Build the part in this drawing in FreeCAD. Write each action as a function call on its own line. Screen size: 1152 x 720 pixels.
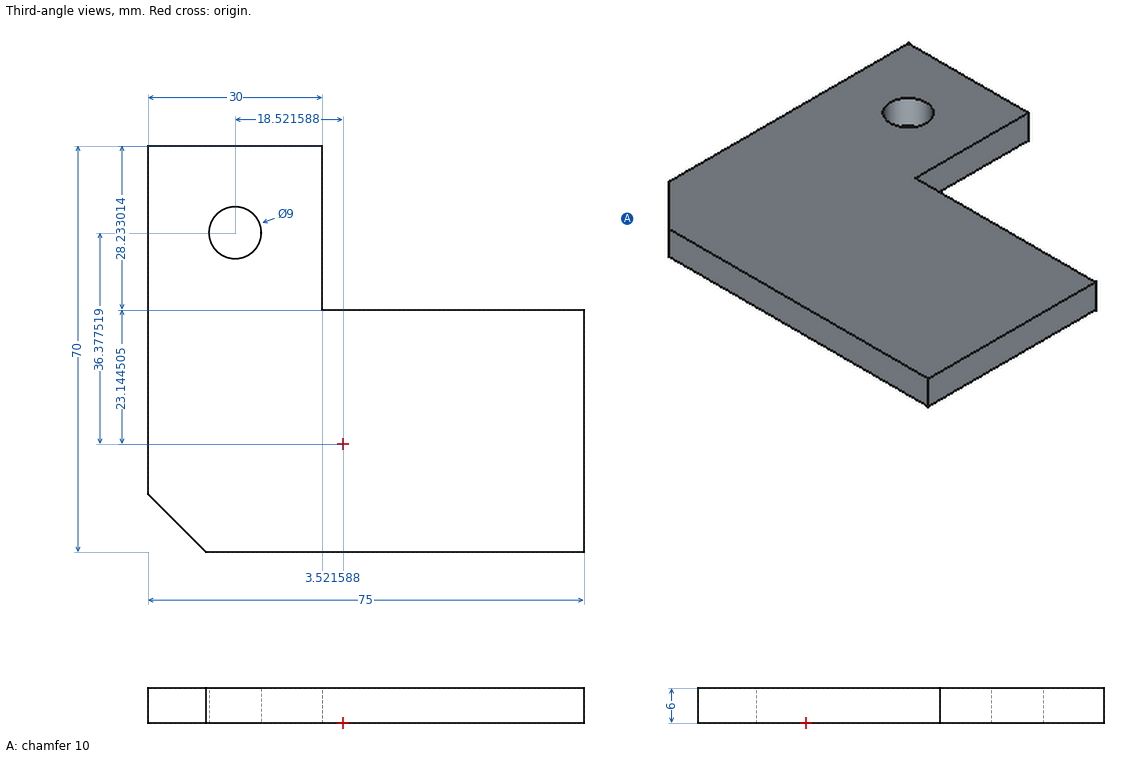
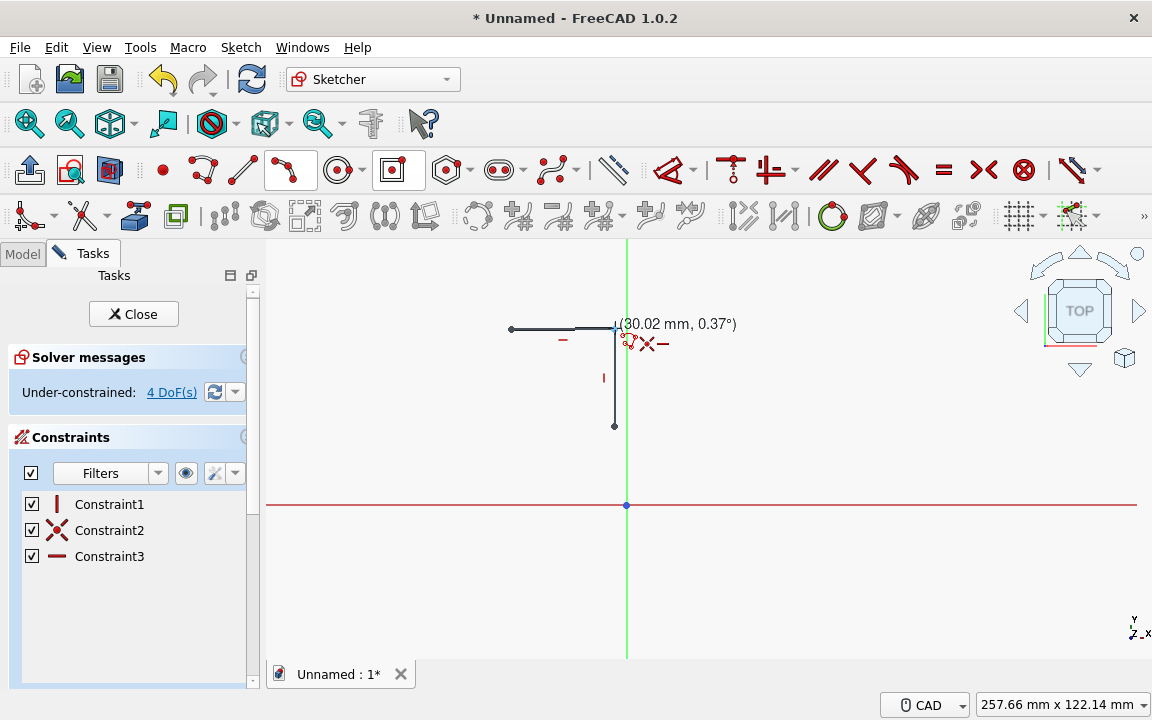
click(512, 569)
click(769, 569)
click(769, 426)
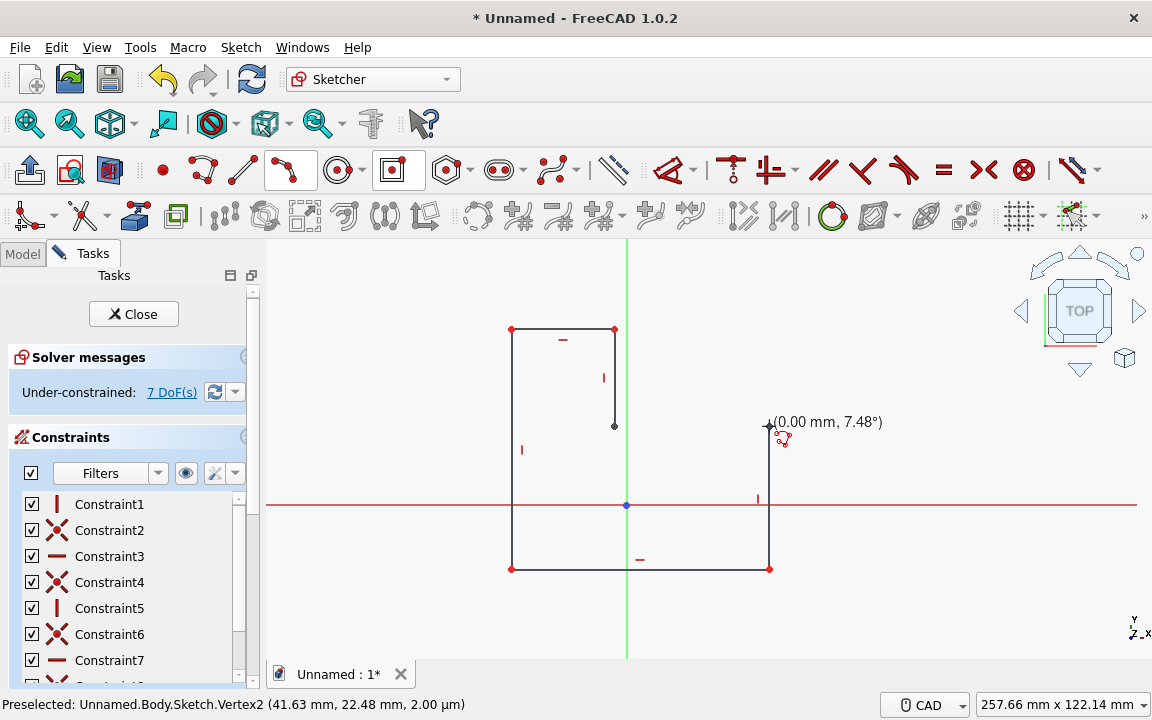
scroll(615, 426, up, 2)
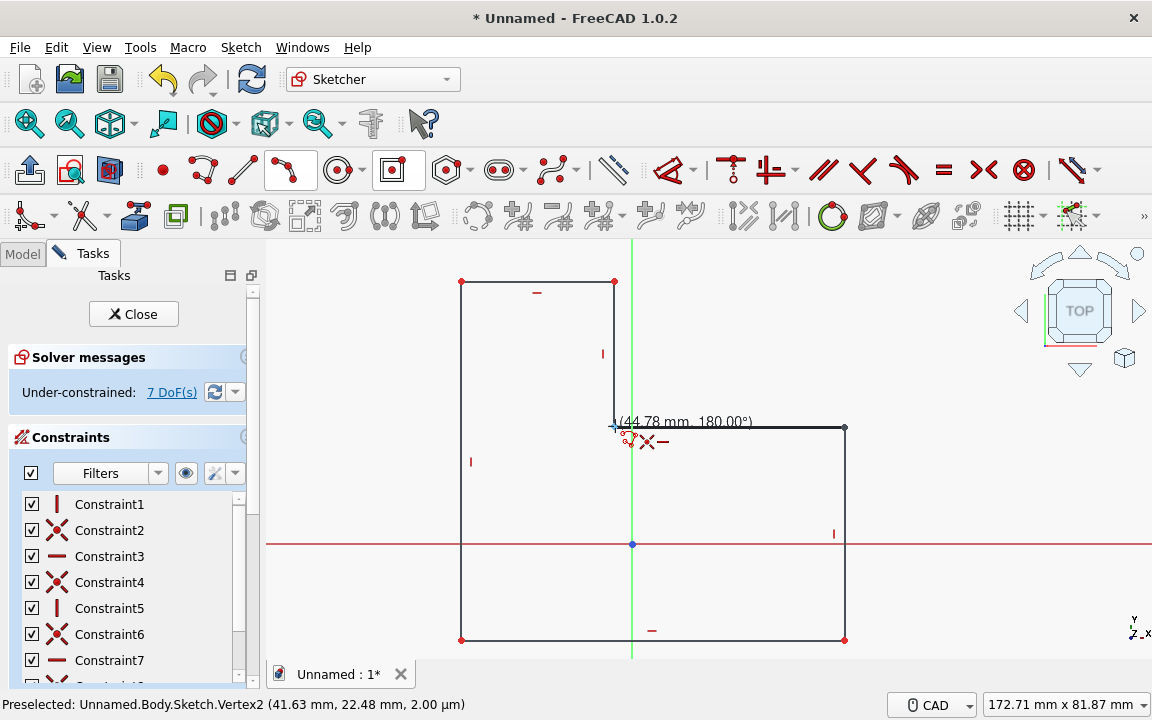
click(614, 426)
key(Escape)
key(Escape)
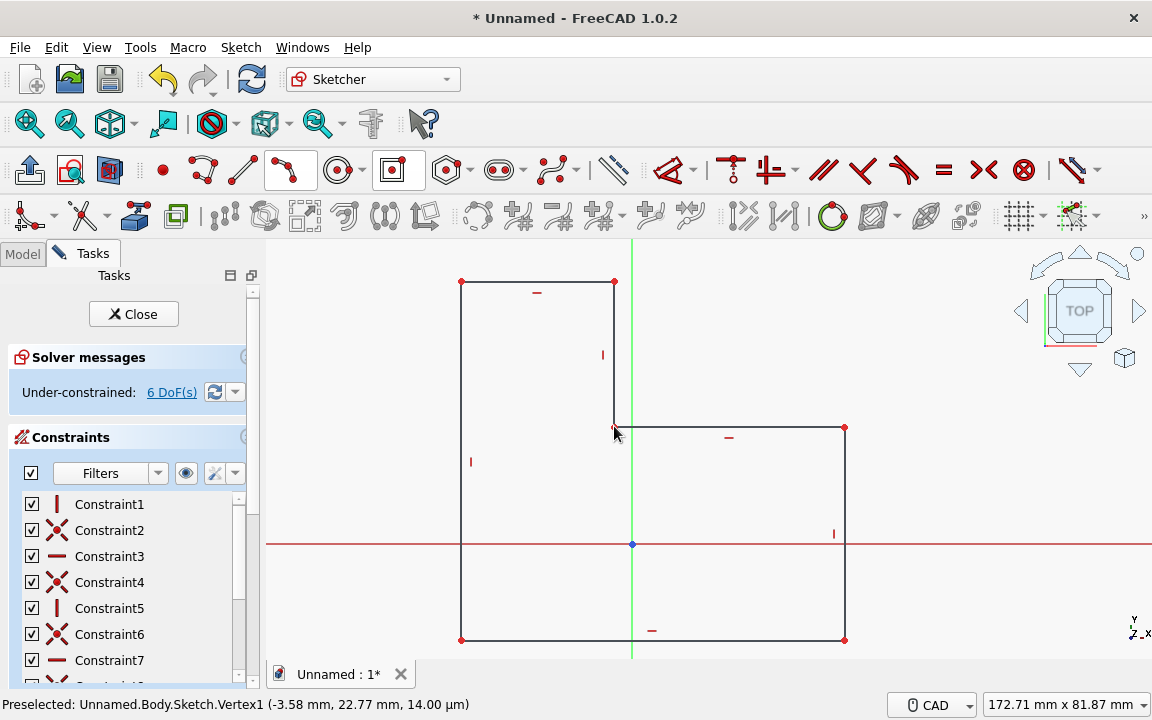
click(568, 282)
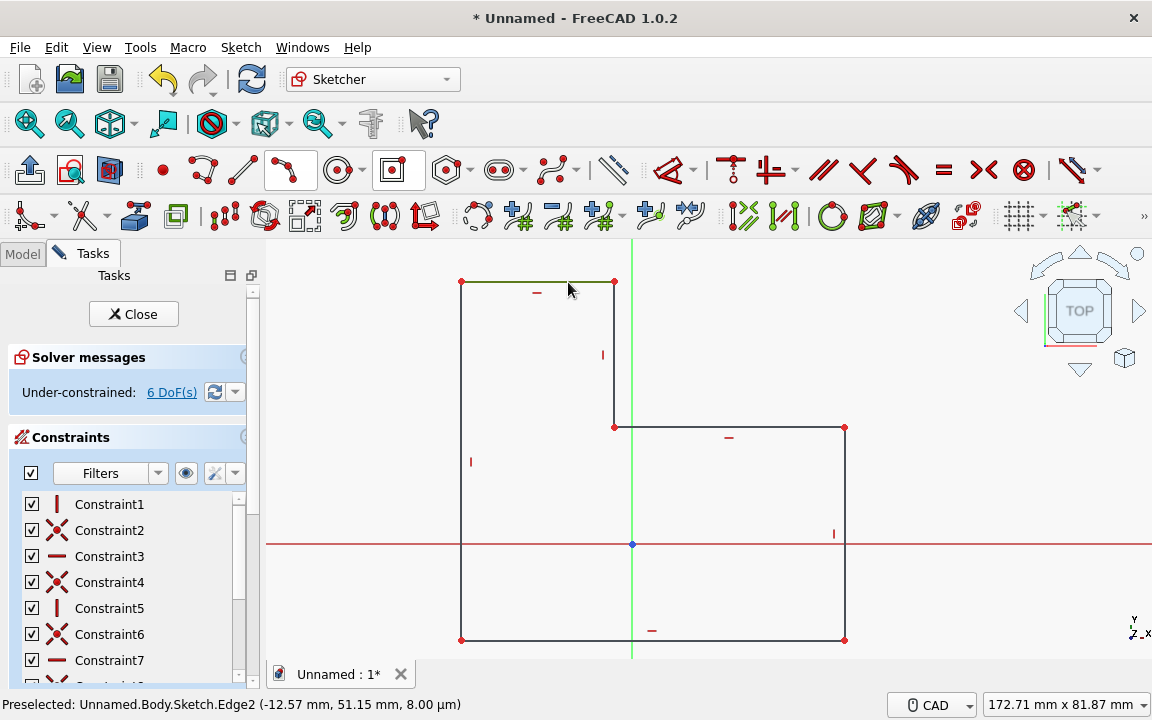
click(696, 170)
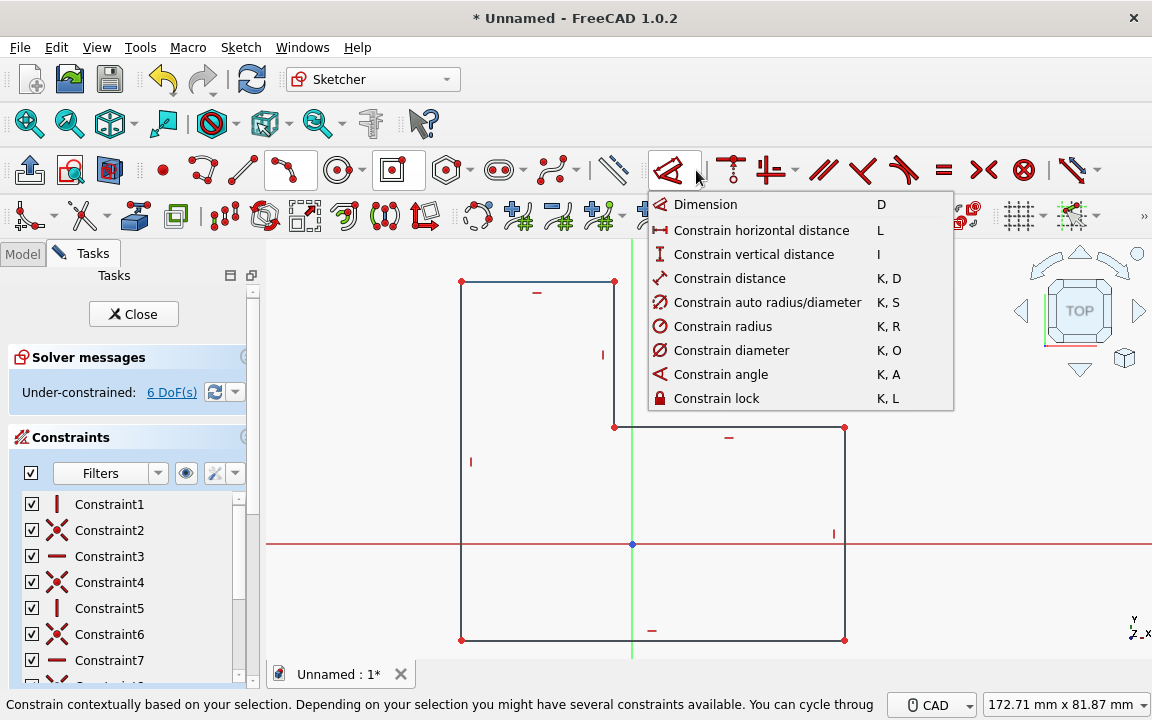
click(801, 230)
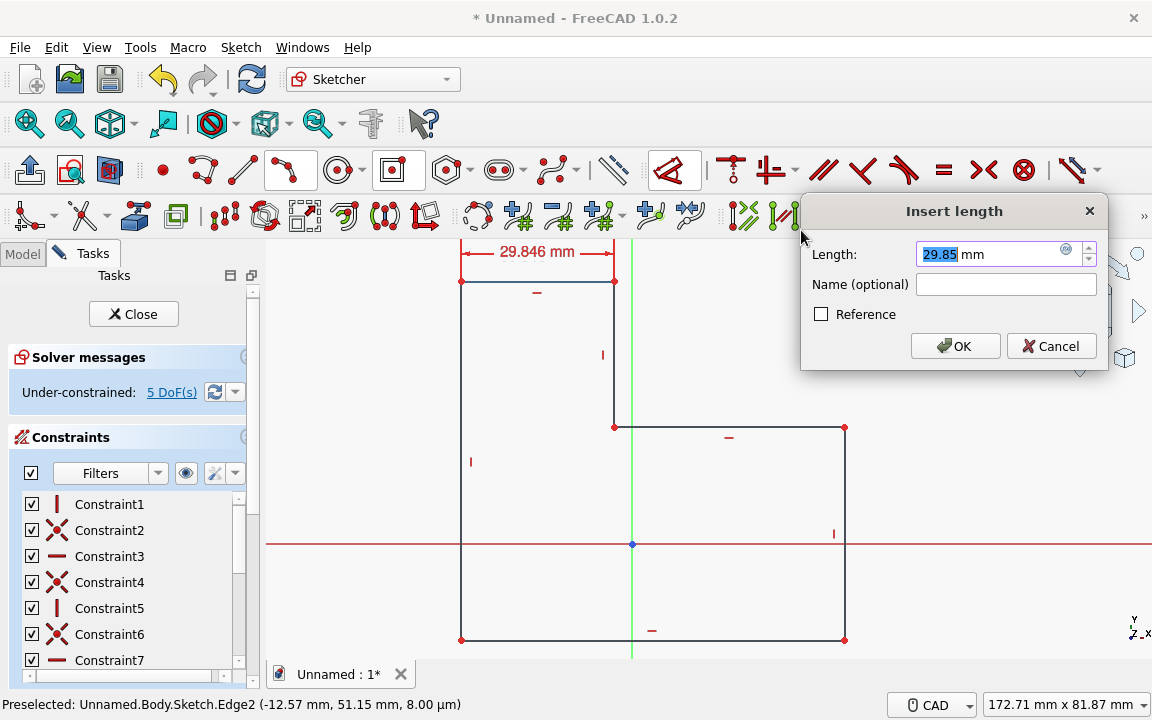
text(30)
key(Return)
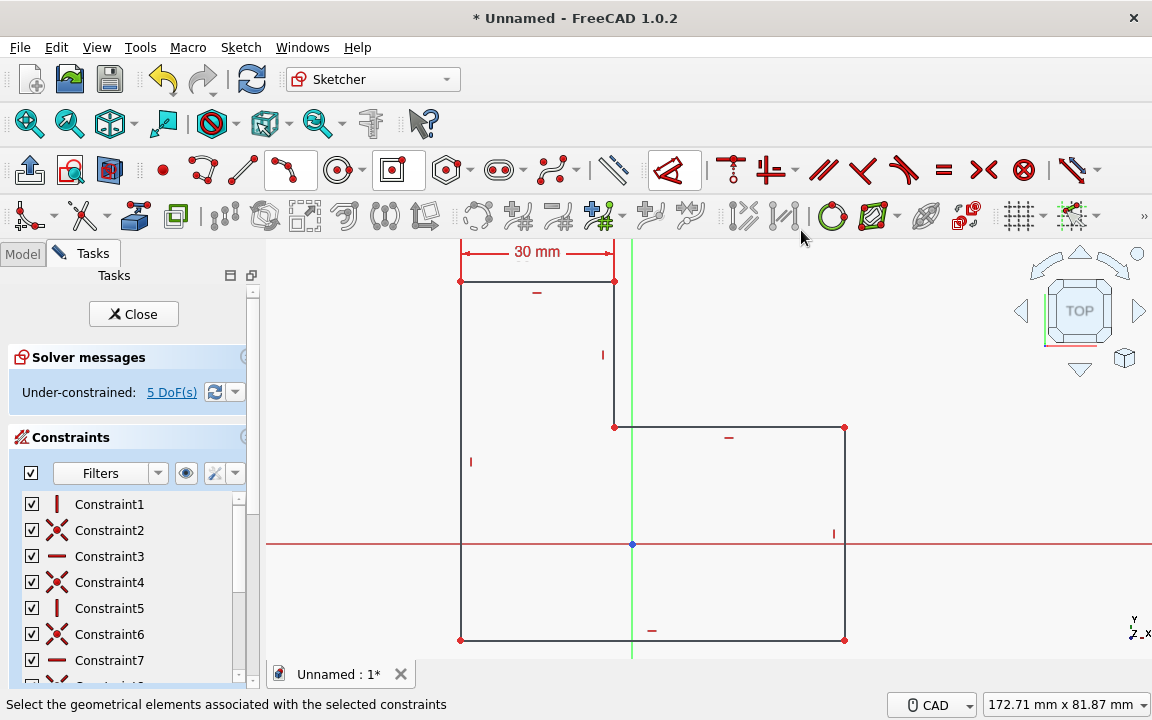
click(461, 389)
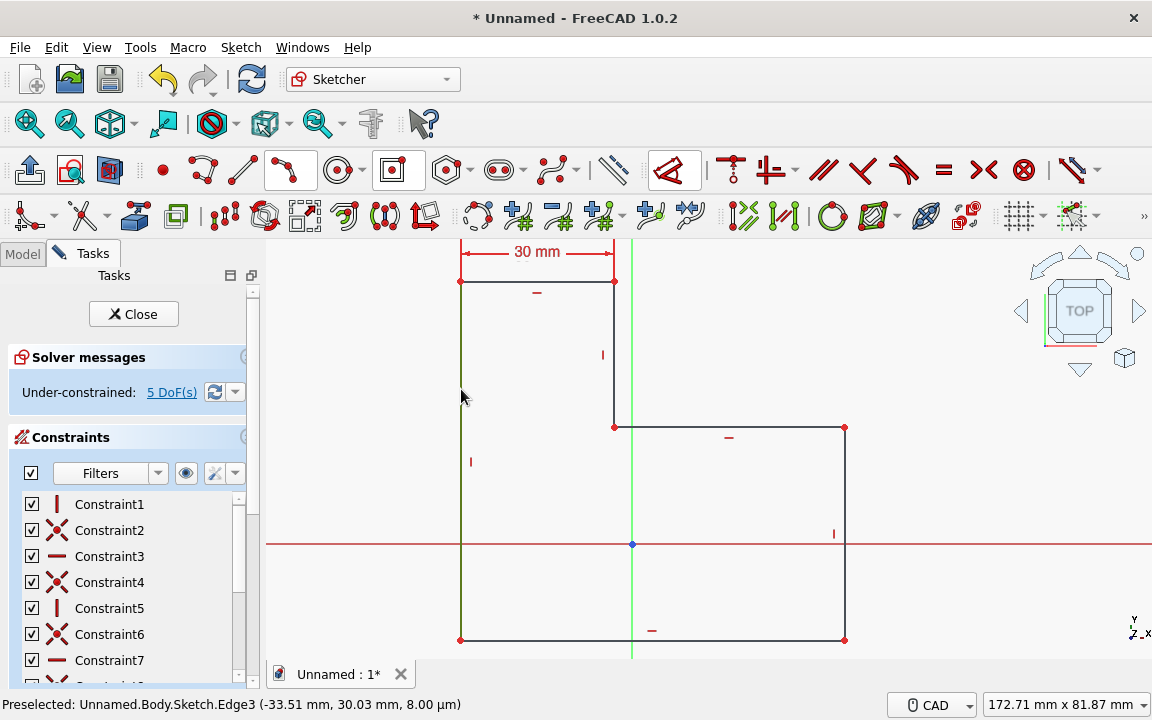
click(696, 170)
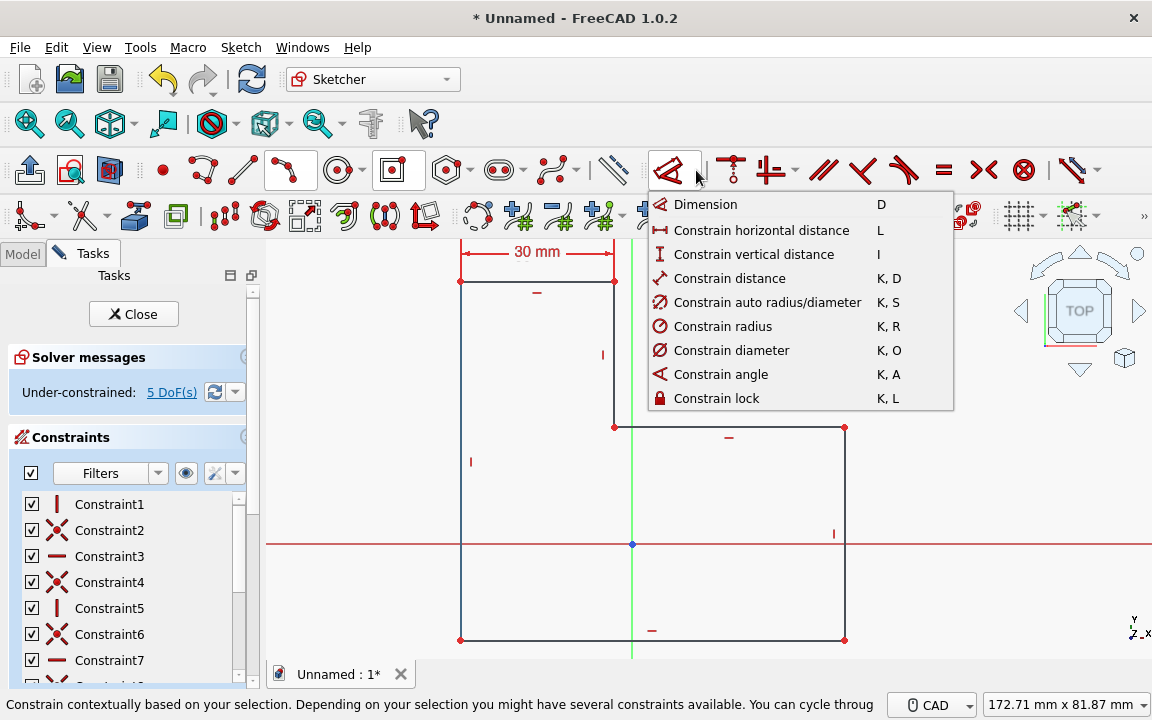
click(801, 254)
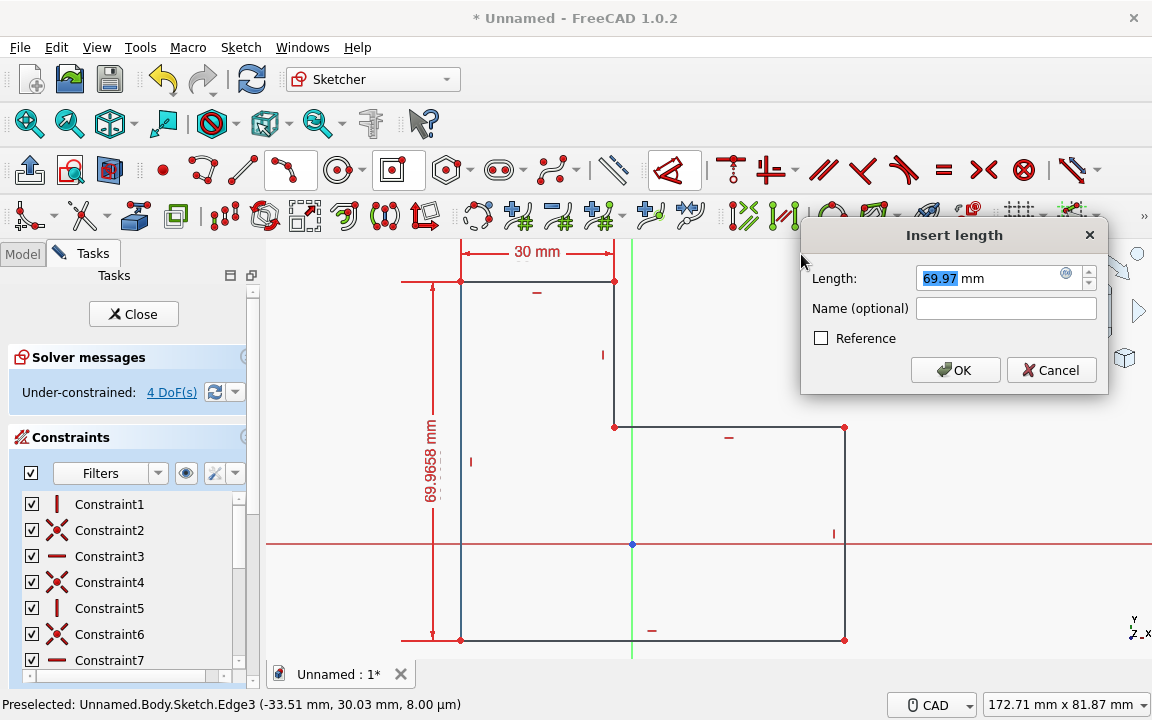
text(70)
key(Return)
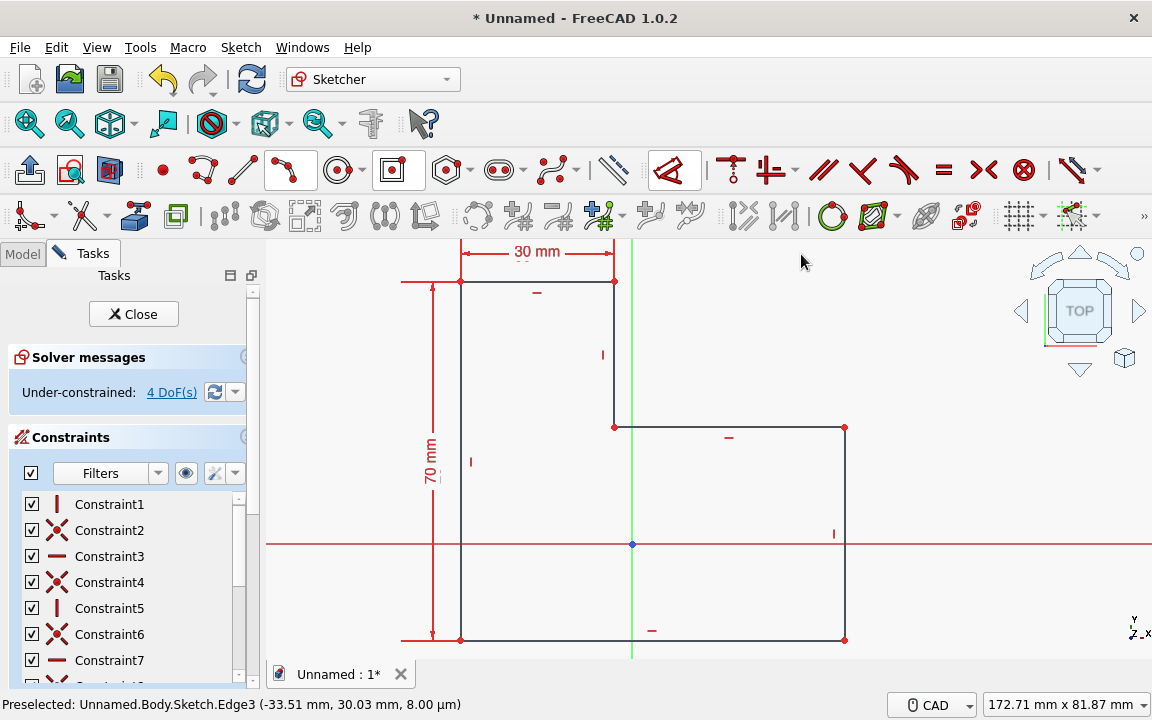
scroll(615, 427, down, 2)